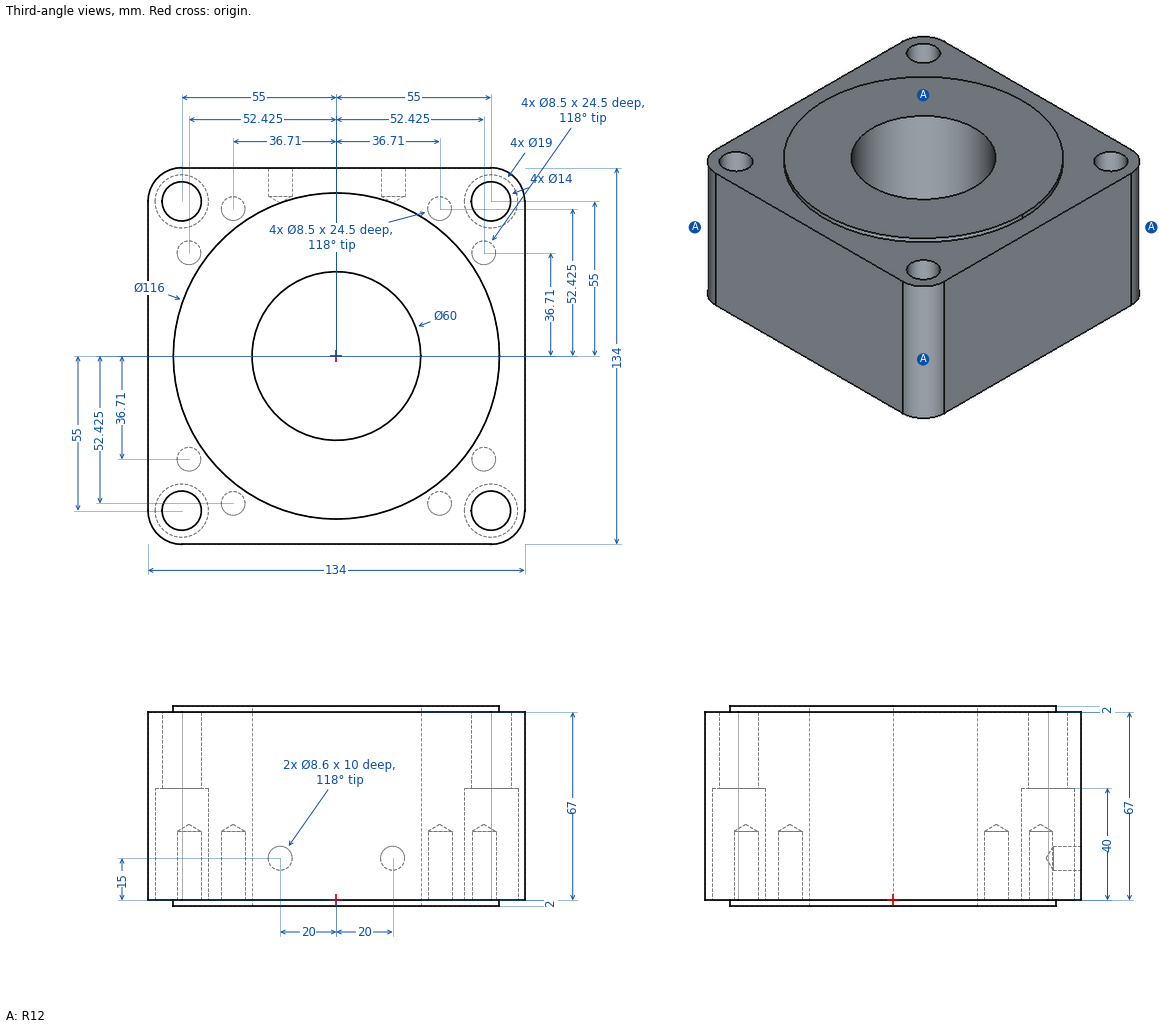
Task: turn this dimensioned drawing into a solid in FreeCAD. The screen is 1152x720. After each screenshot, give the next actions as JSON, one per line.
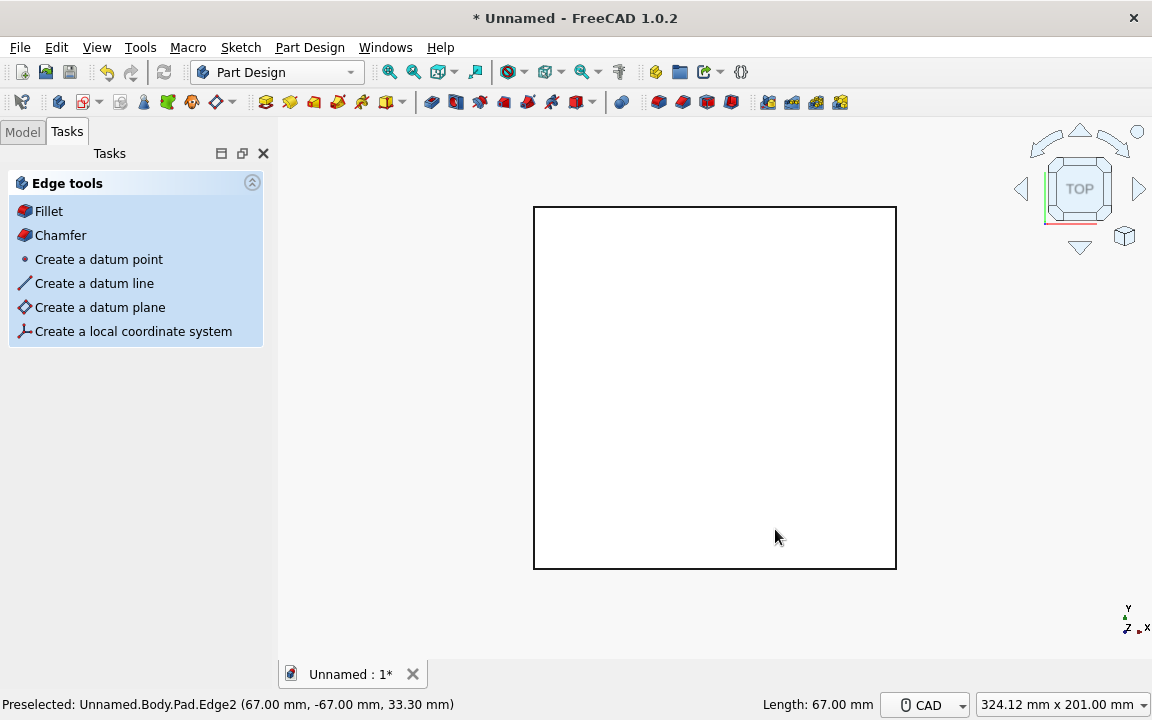
{"action": "key", "text": "1"}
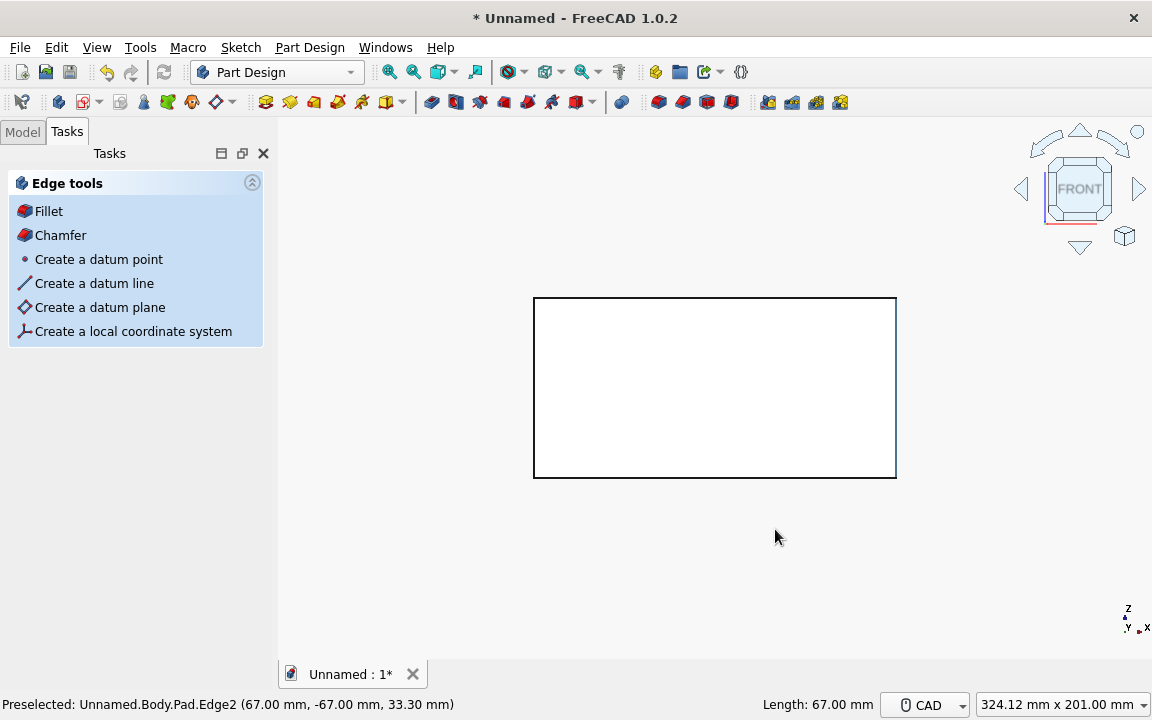
{"action": "left_click", "coordinate": [390, 72]}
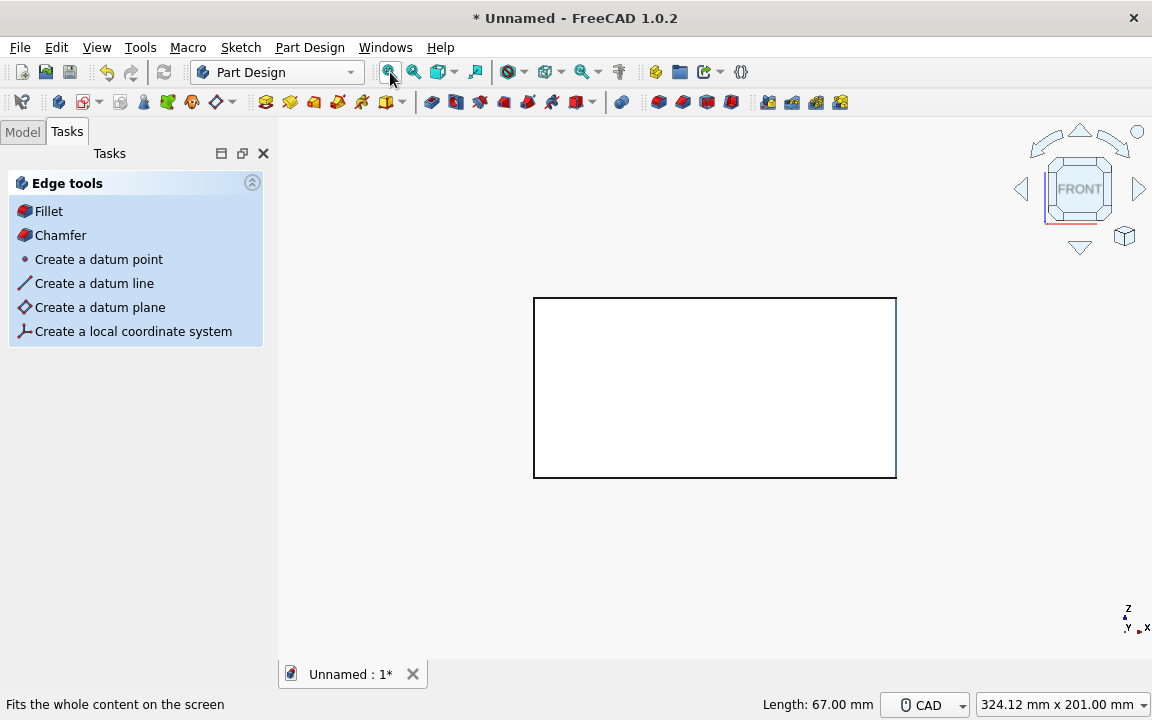
{"action": "left_click", "coordinate": [534, 387], "text": "ctrl"}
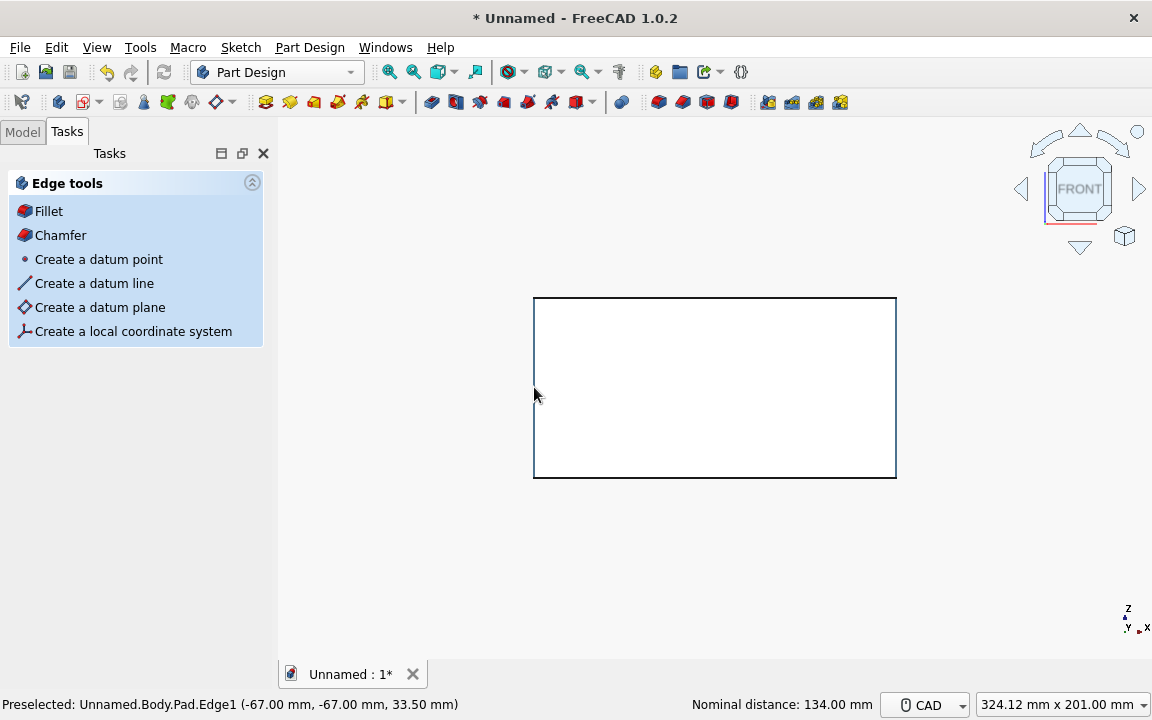
{"action": "key", "text": "3"}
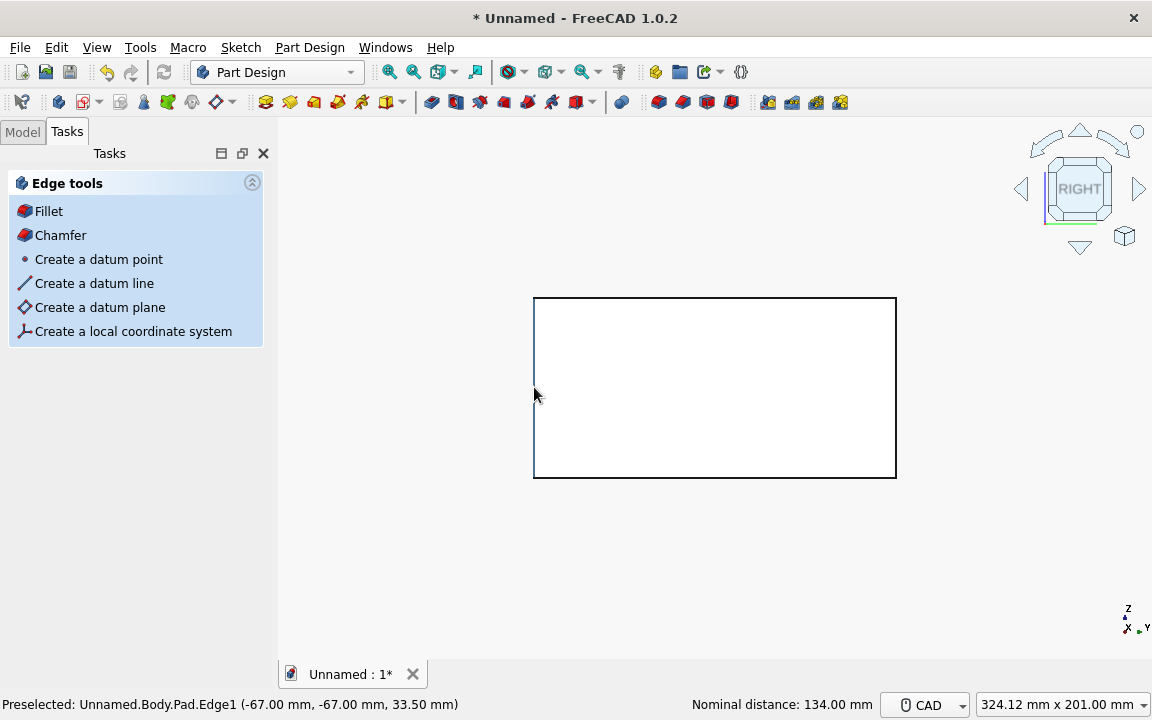
{"action": "left_click", "coordinate": [390, 72]}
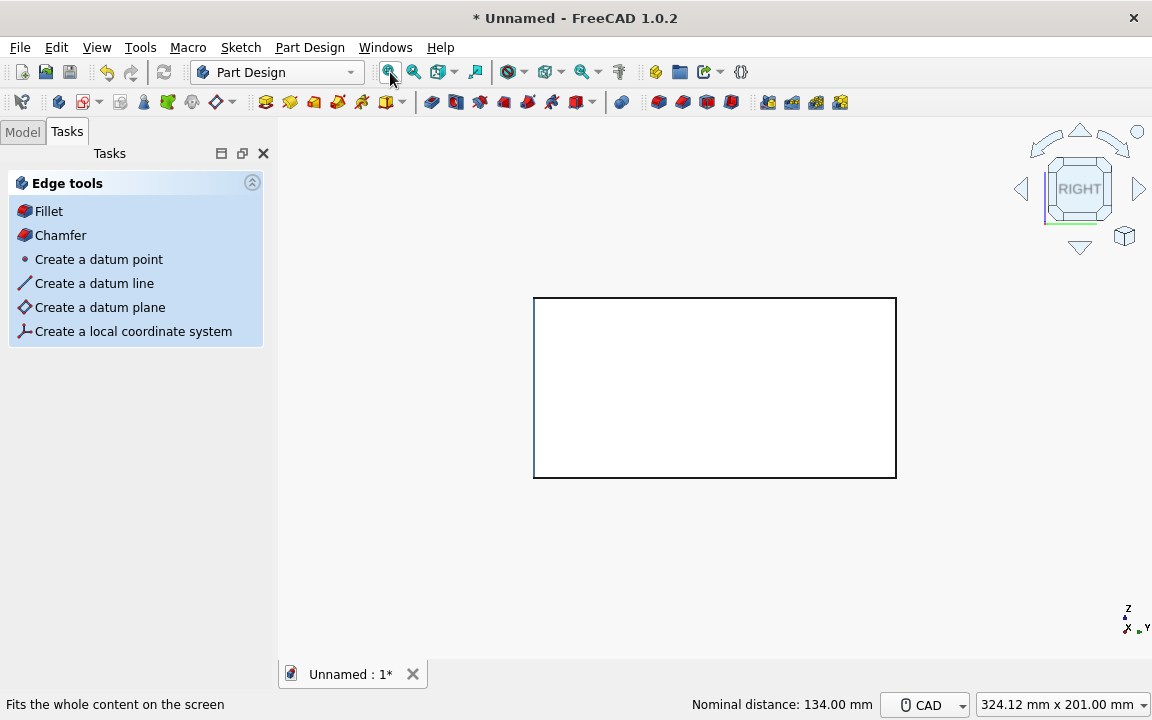
{"action": "left_click", "coordinate": [896, 387], "text": "ctrl"}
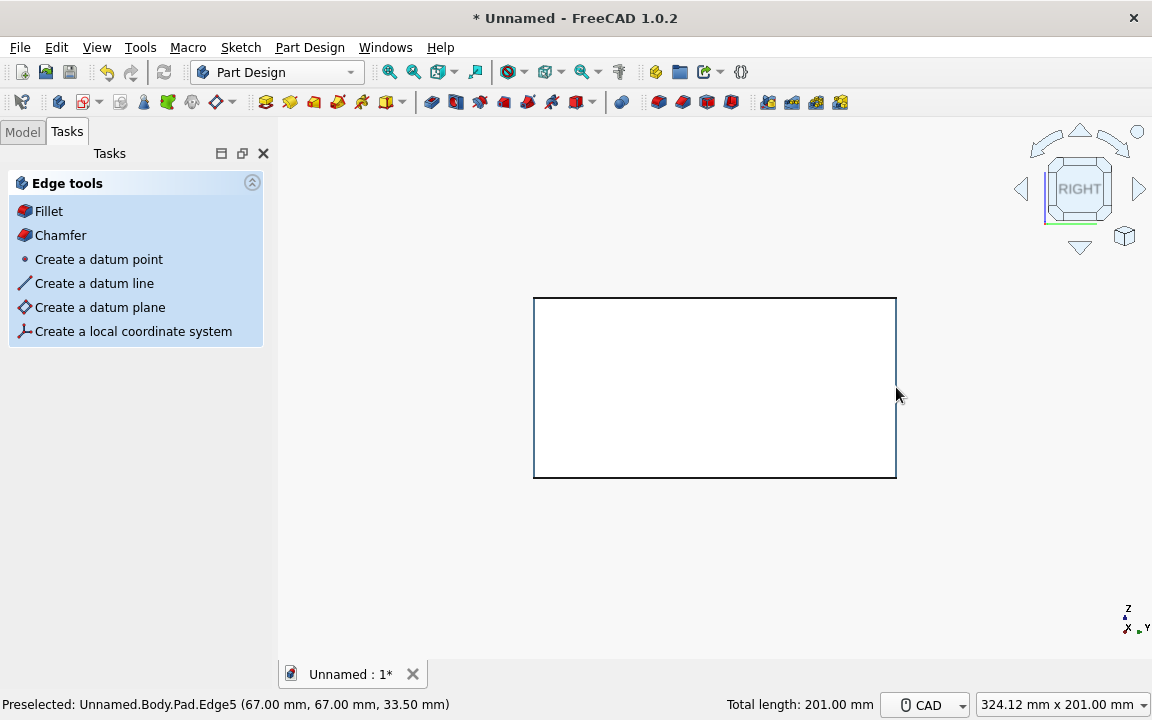
{"action": "key", "text": "5"}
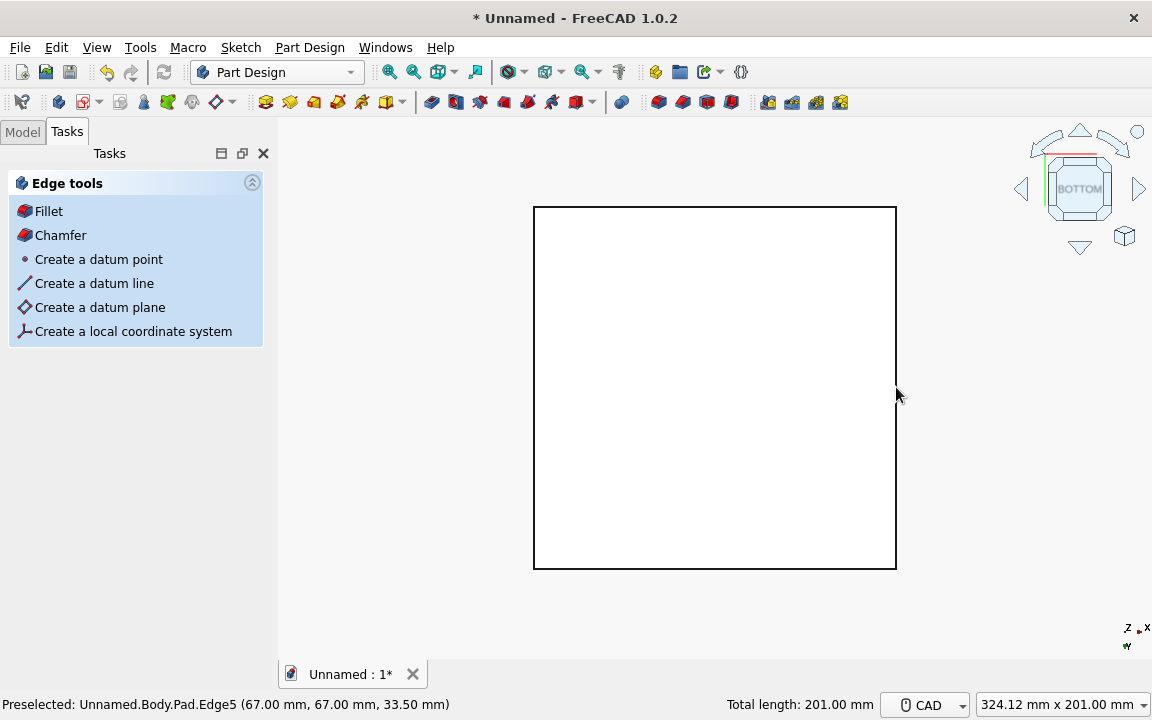
{"action": "key", "text": "4"}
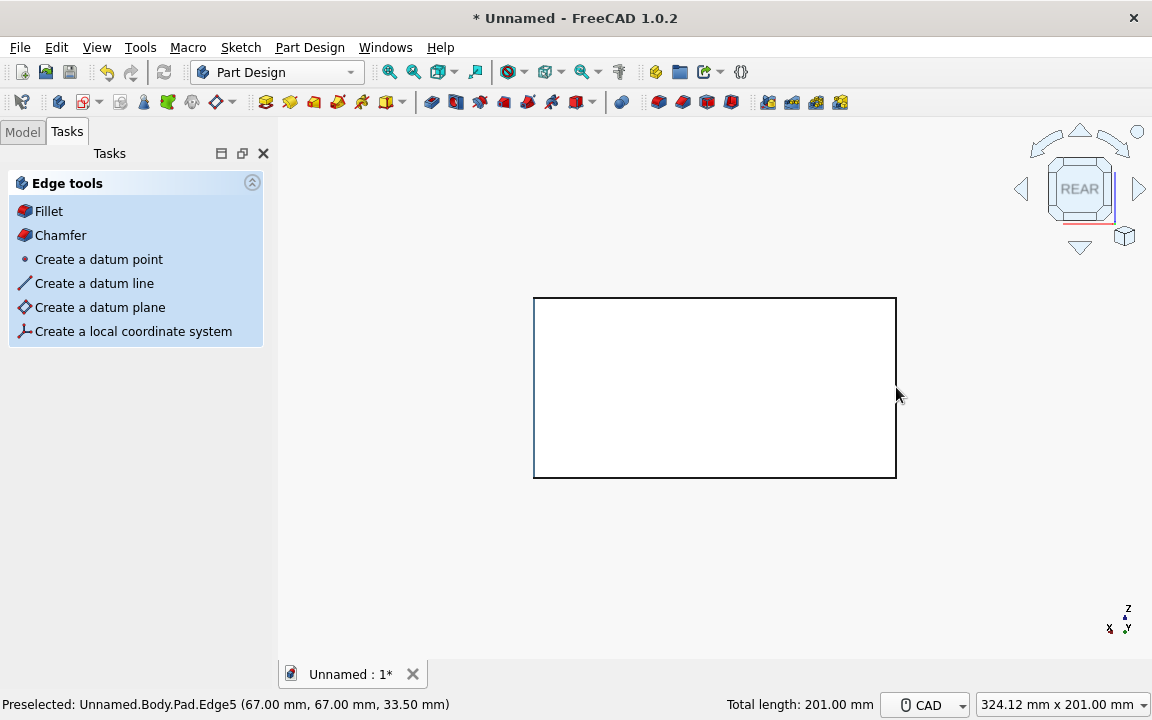
{"action": "left_click", "coordinate": [390, 72]}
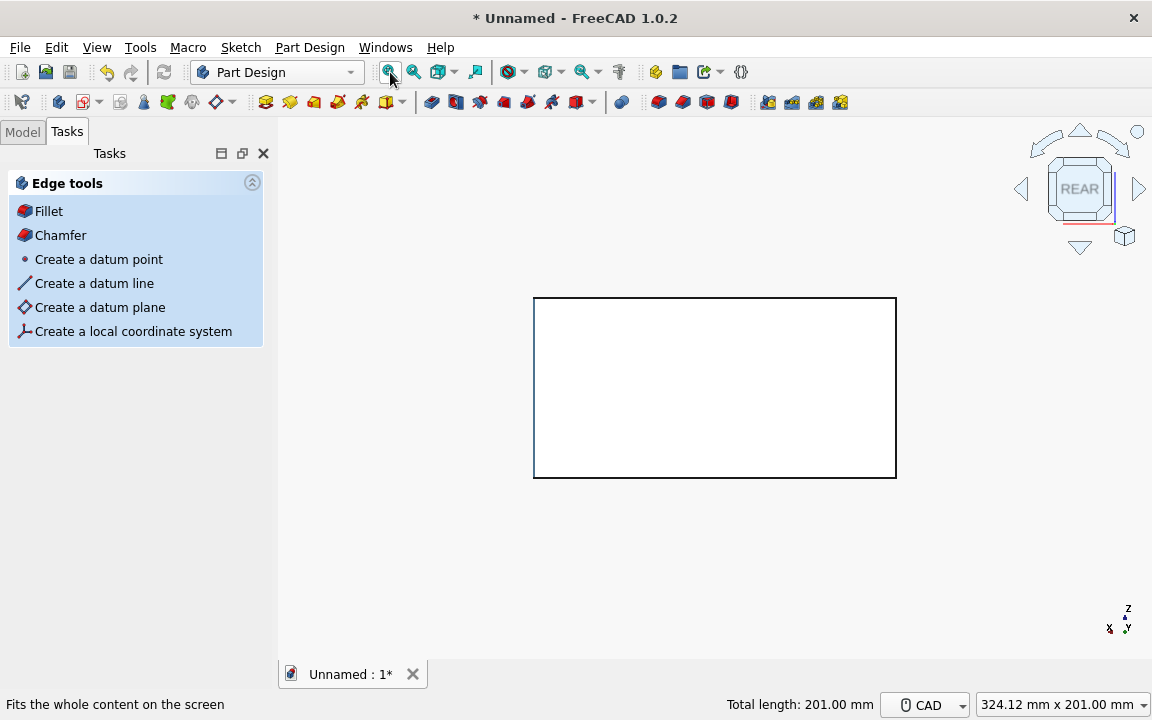
{"action": "left_click", "coordinate": [896, 387], "text": "ctrl"}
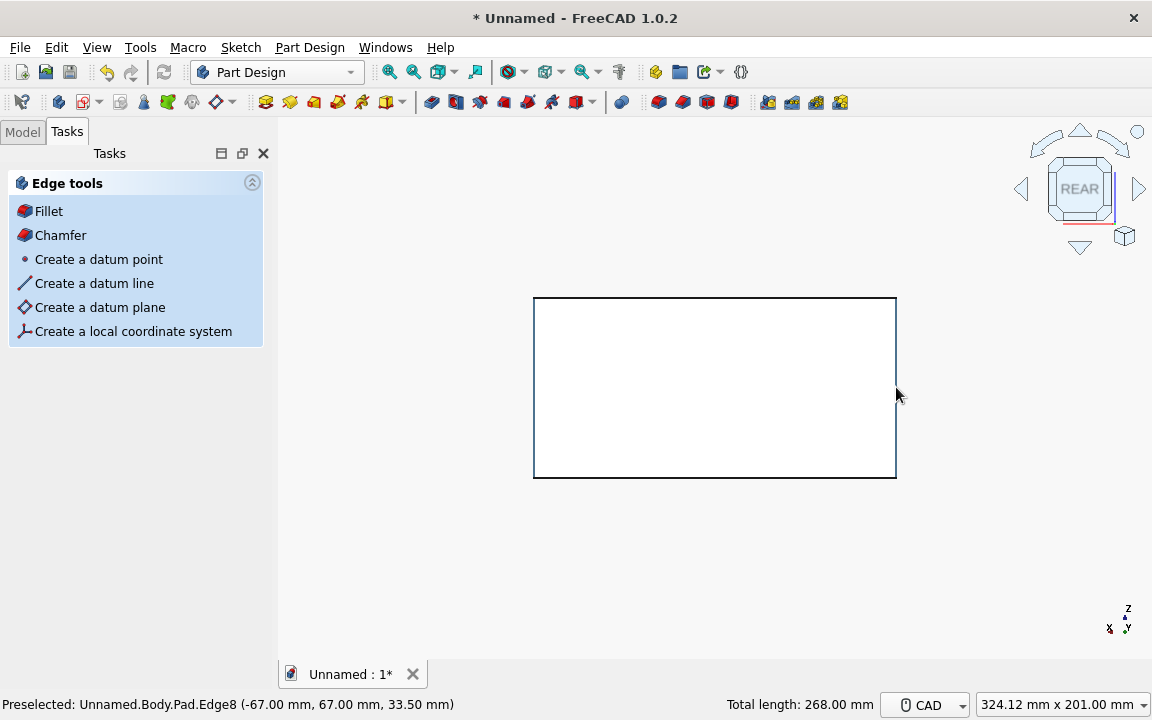
{"action": "left_click", "coordinate": [660, 102]}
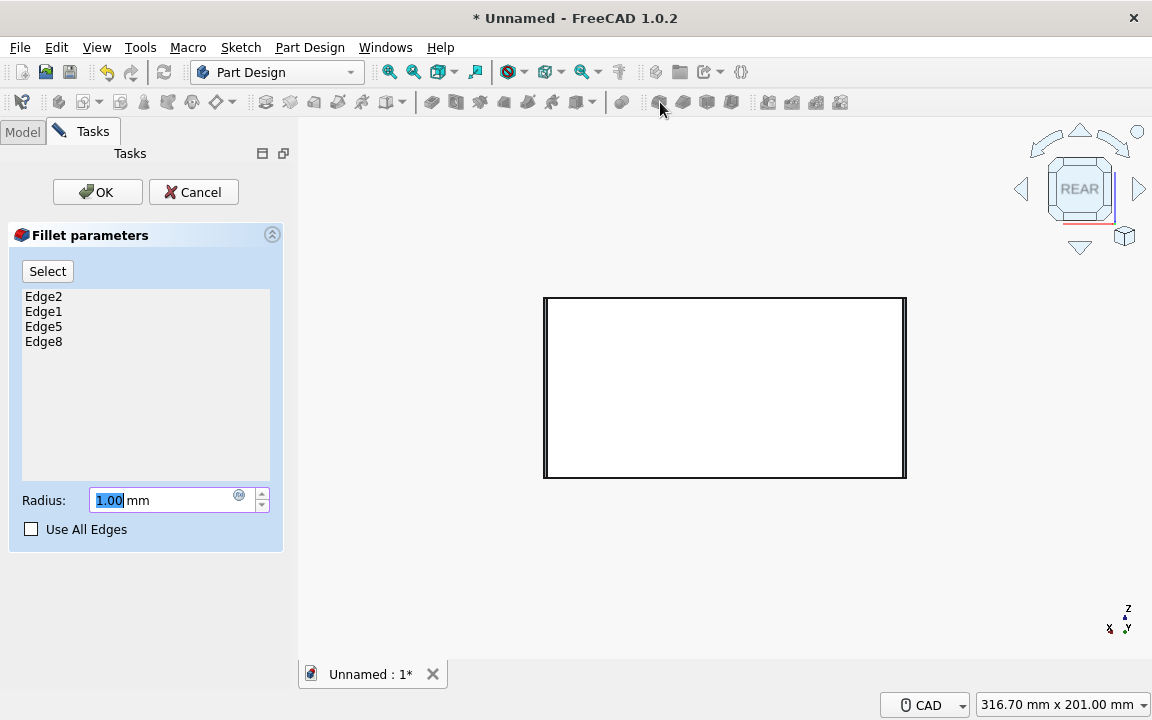
{"action": "type", "text": "12"}
{"action": "key", "text": "Tab"}